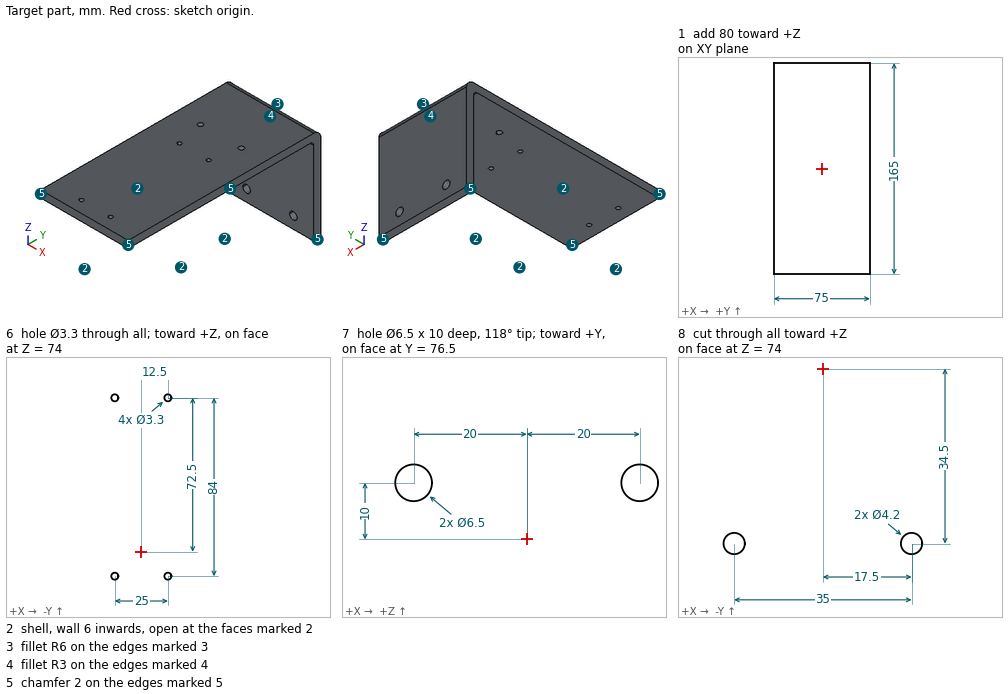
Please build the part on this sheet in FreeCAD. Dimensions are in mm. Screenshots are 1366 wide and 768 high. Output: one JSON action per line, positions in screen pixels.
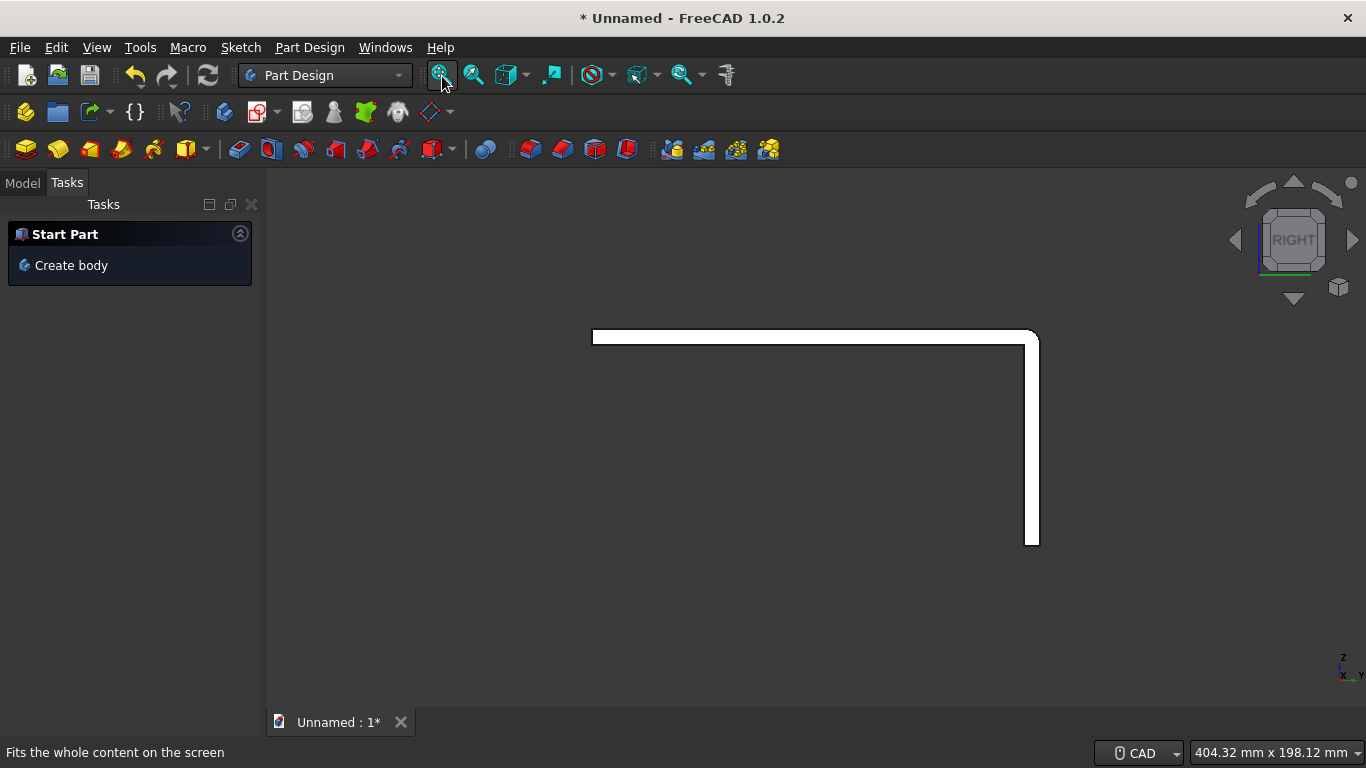
{"action": "key", "text": "5"}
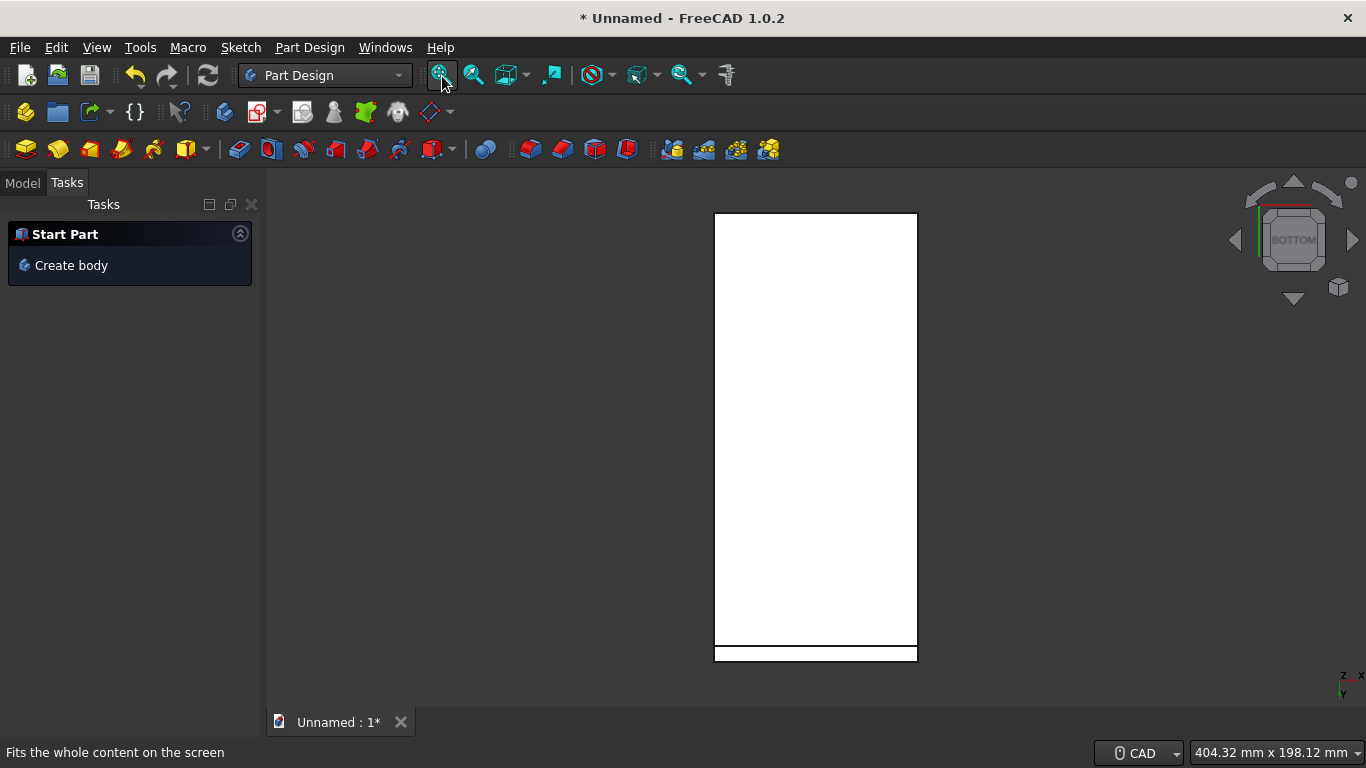
{"action": "key", "text": "4"}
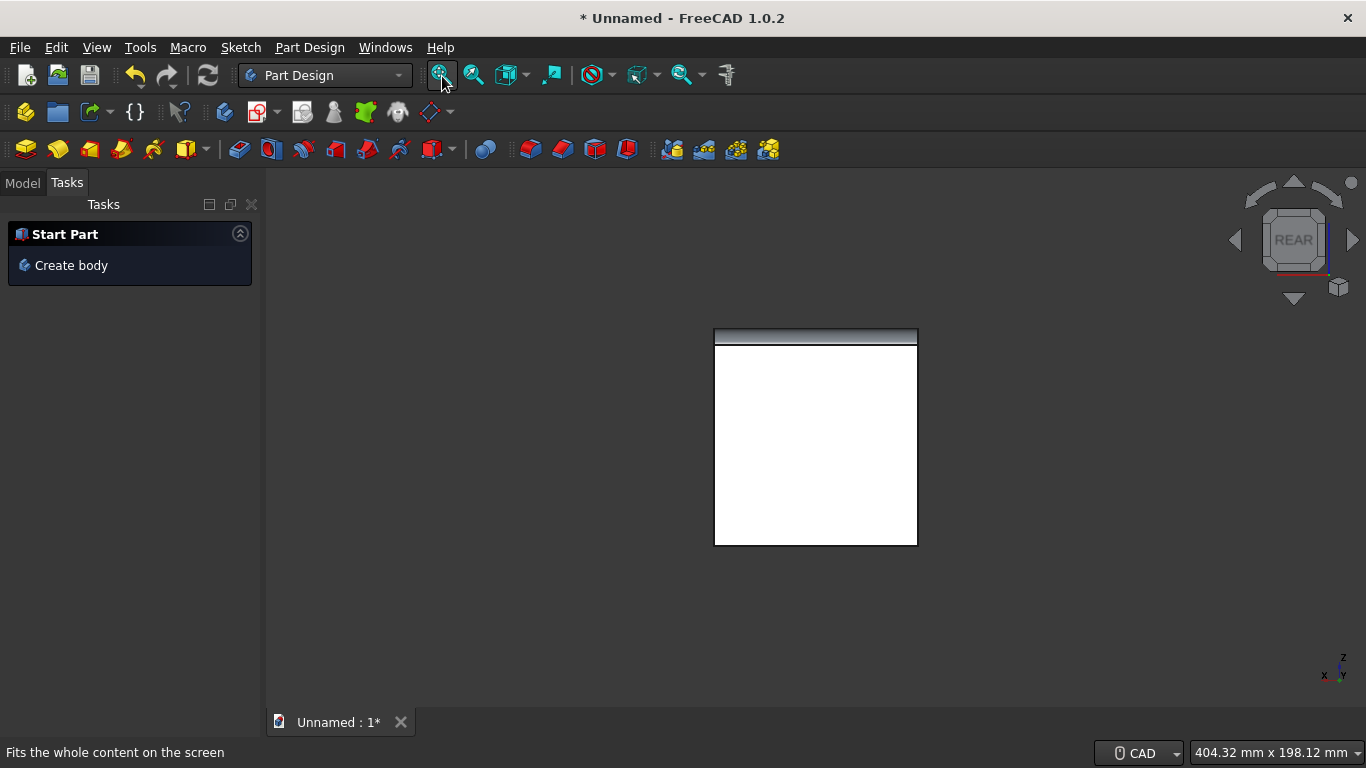
{"action": "left_click", "coordinate": [442, 76]}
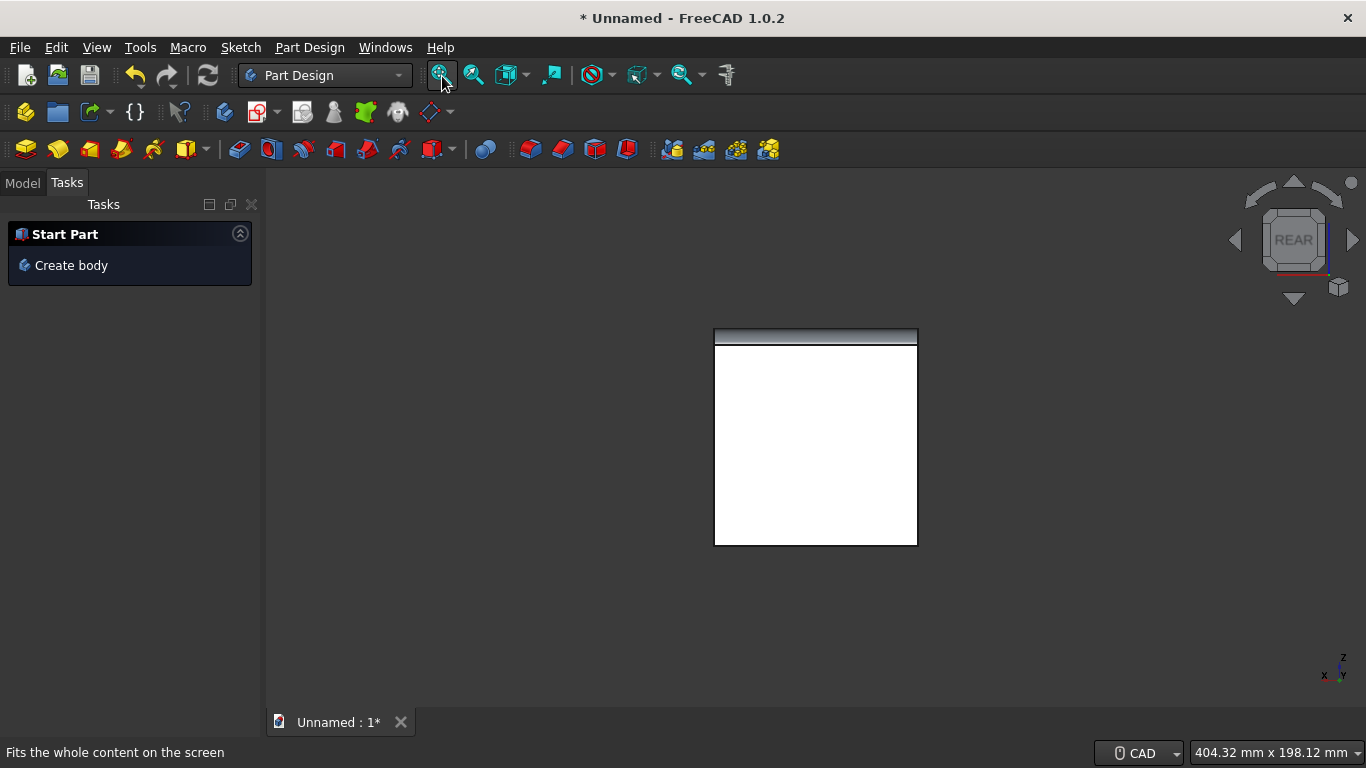
{"action": "key", "text": "6"}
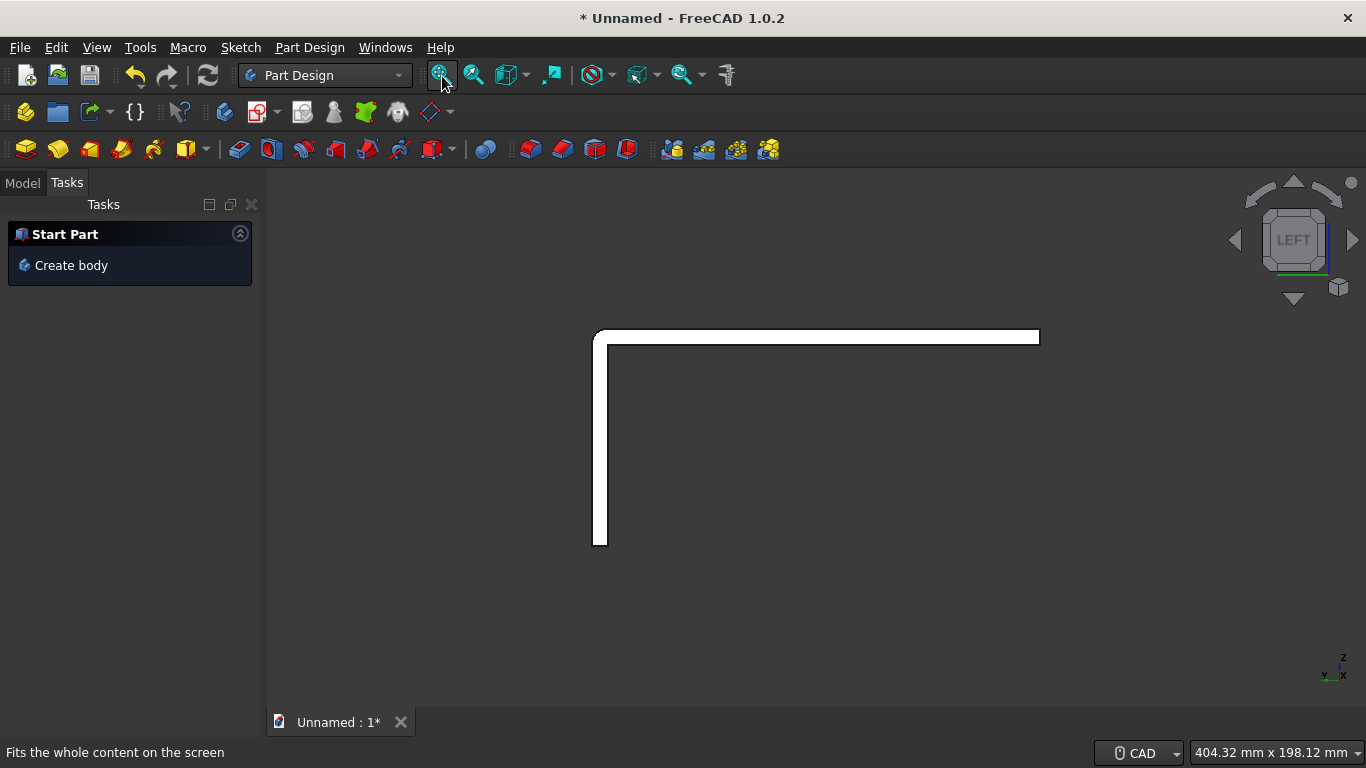
{"action": "left_click", "coordinate": [442, 76]}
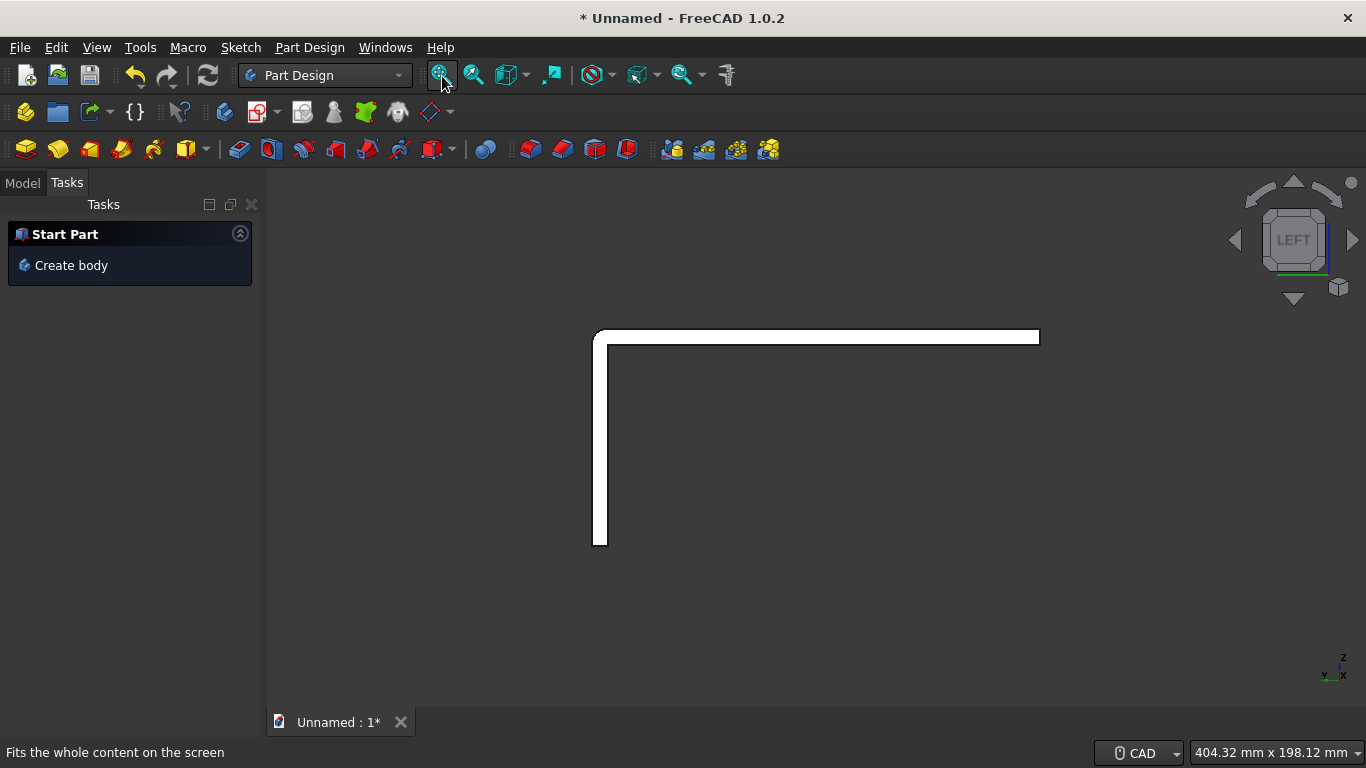
{"action": "key", "text": "v 3"}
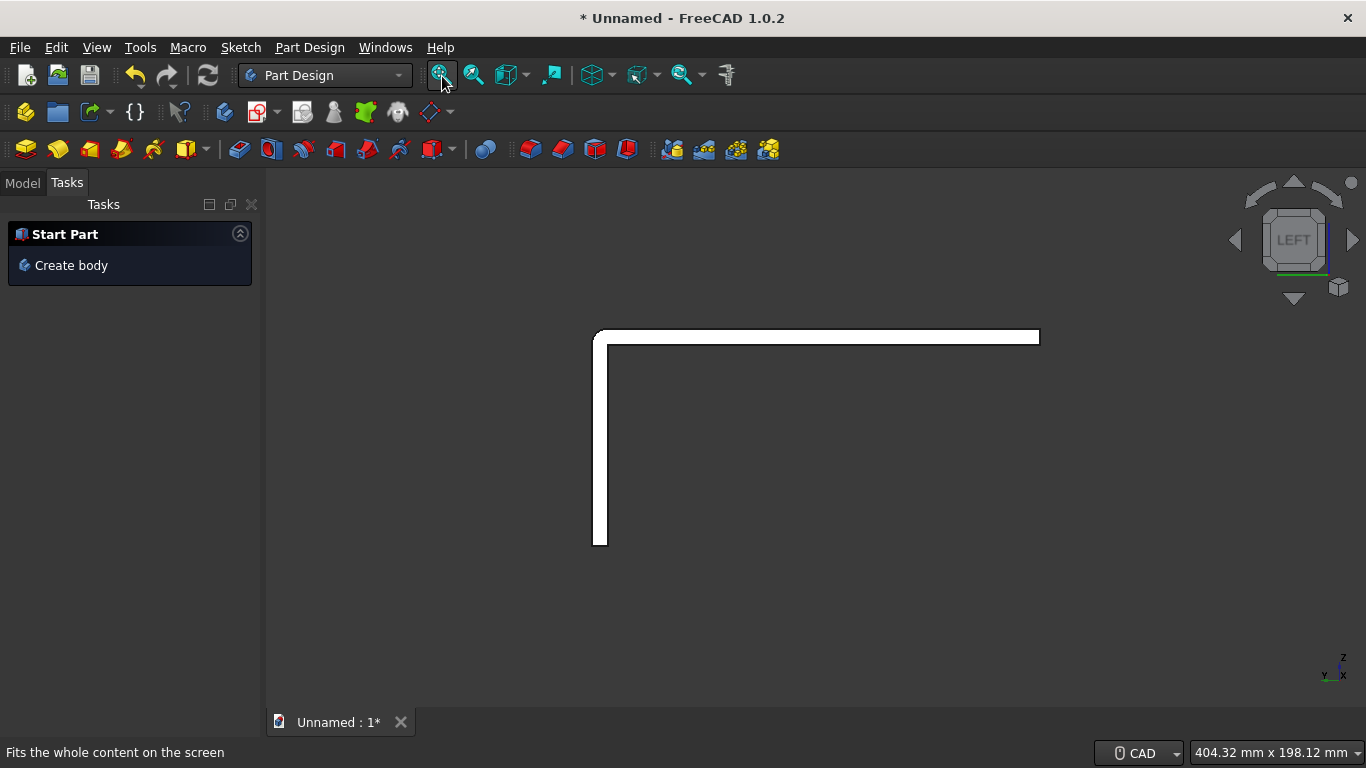
{"action": "key", "text": "0"}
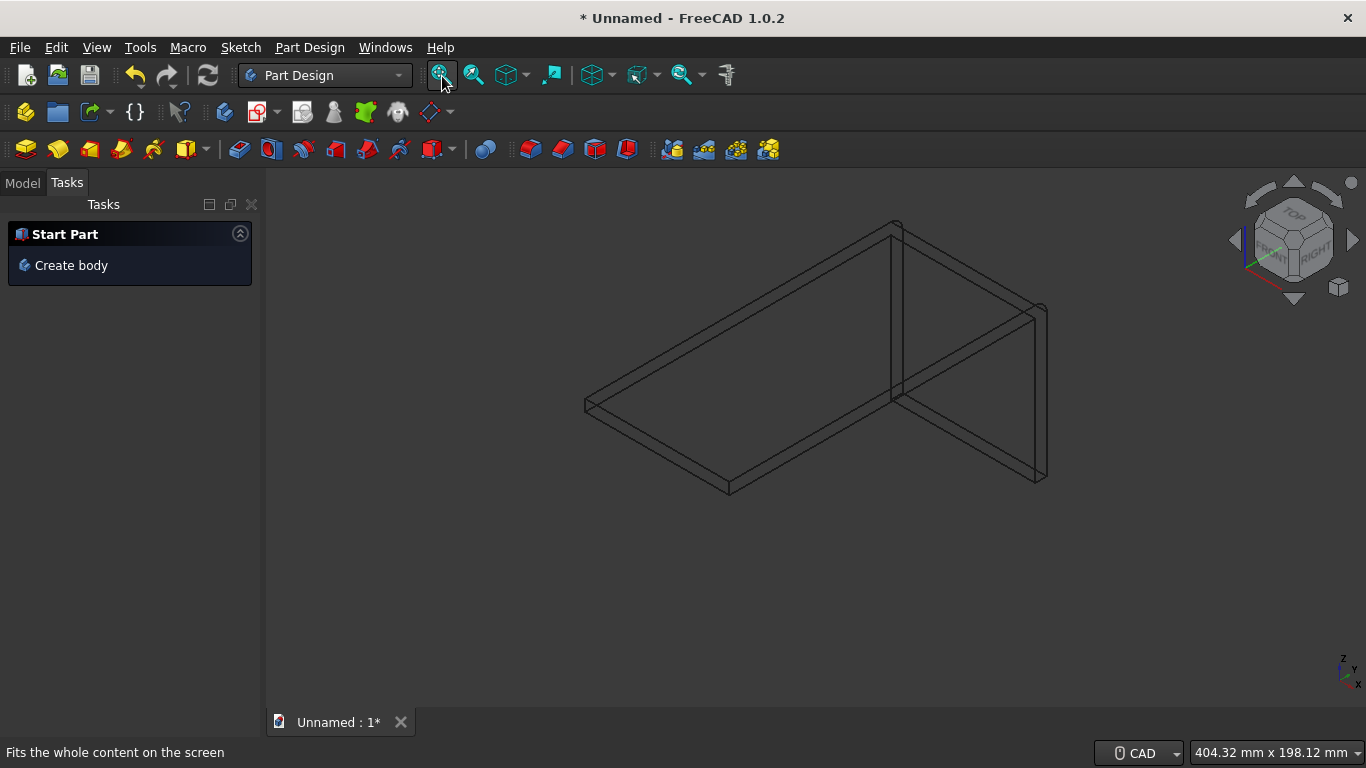
{"action": "left_click", "coordinate": [963, 276]}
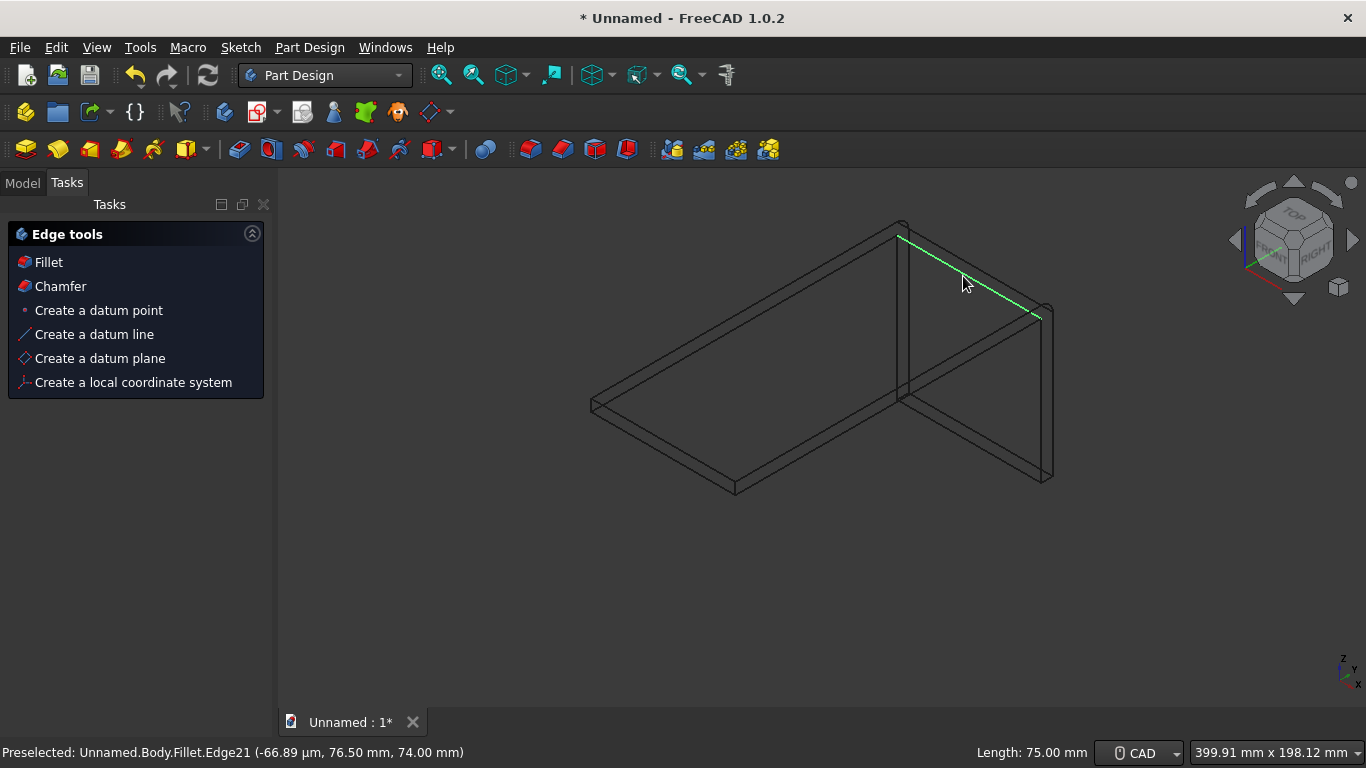
{"action": "key", "text": "v 1"}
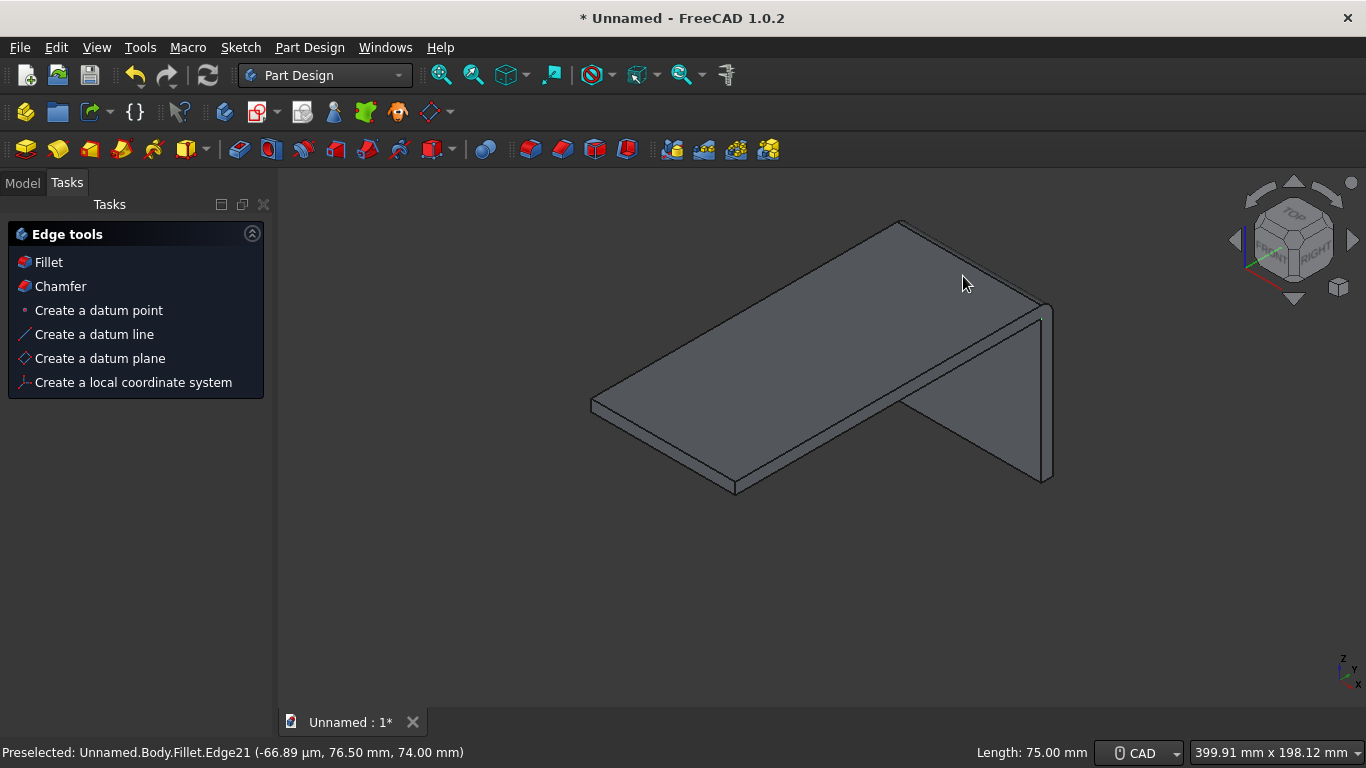
{"action": "left_click", "coordinate": [532, 150]}